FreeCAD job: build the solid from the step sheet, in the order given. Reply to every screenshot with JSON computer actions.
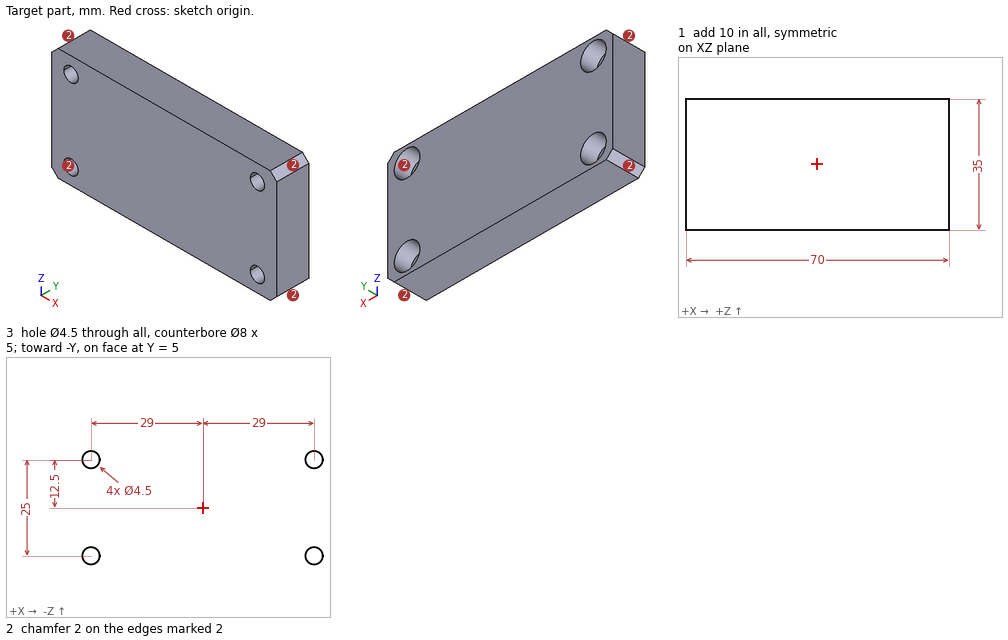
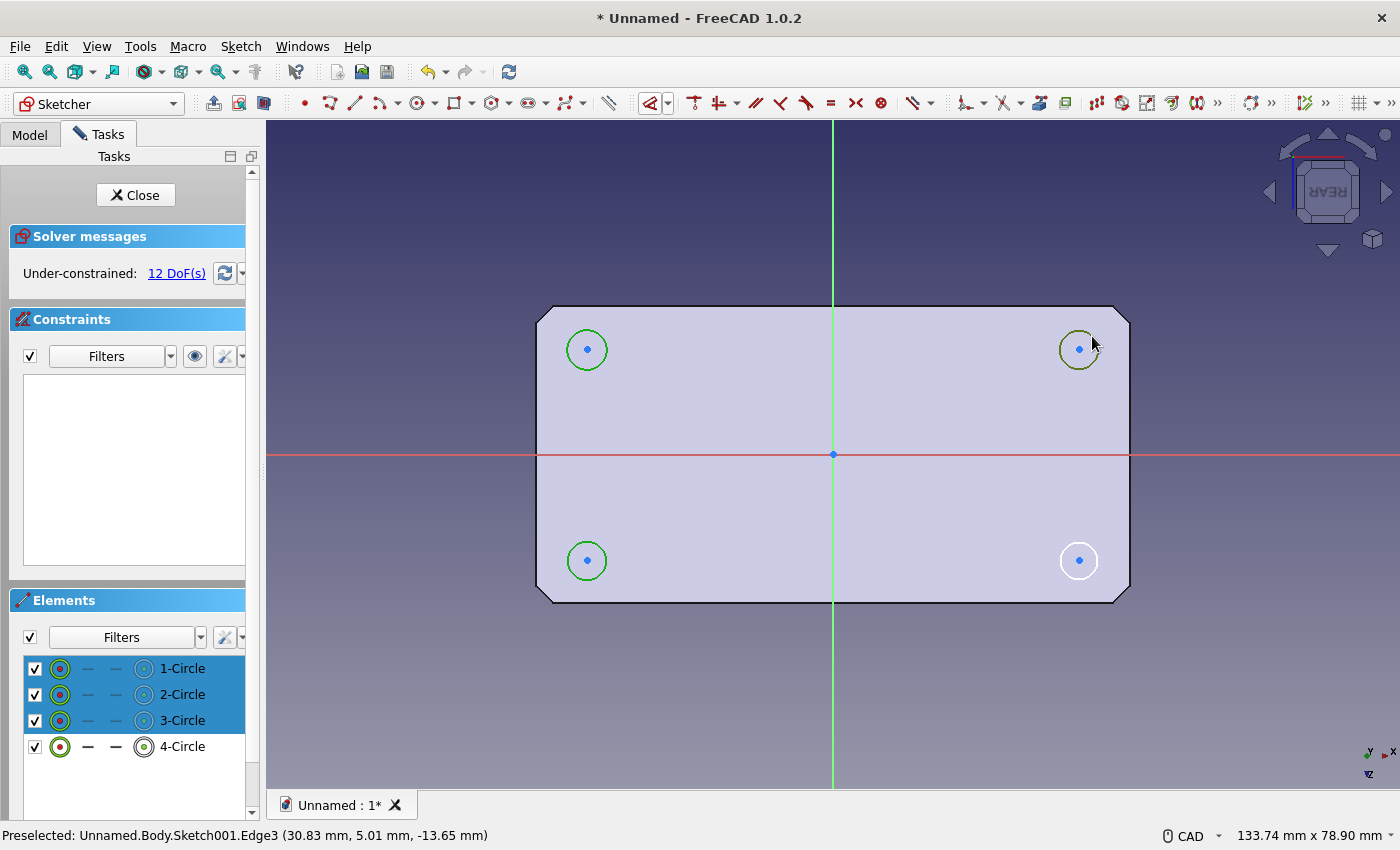
{"action": "left_click", "coordinate": [1092, 548]}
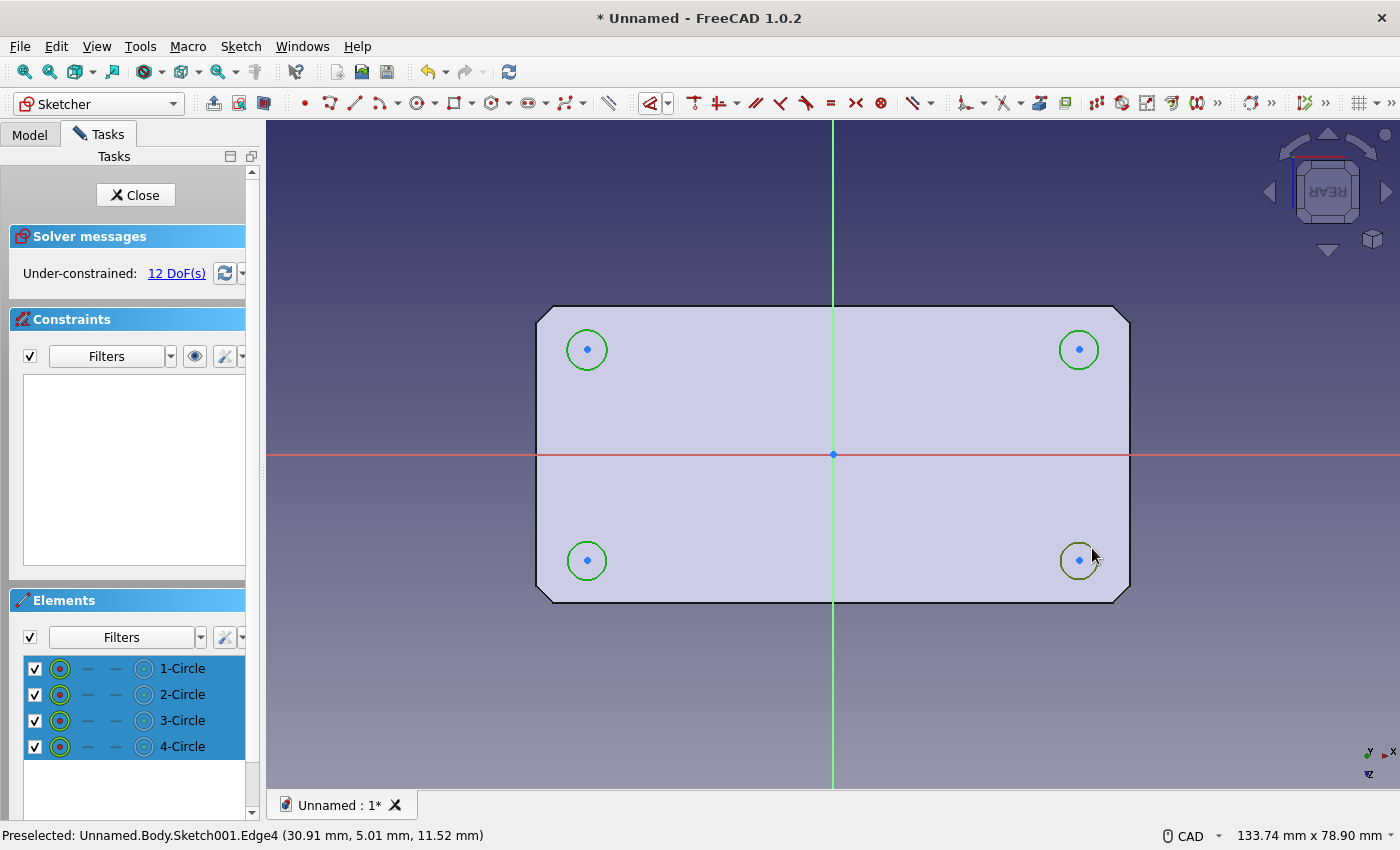
{"action": "left_click", "coordinate": [831, 104]}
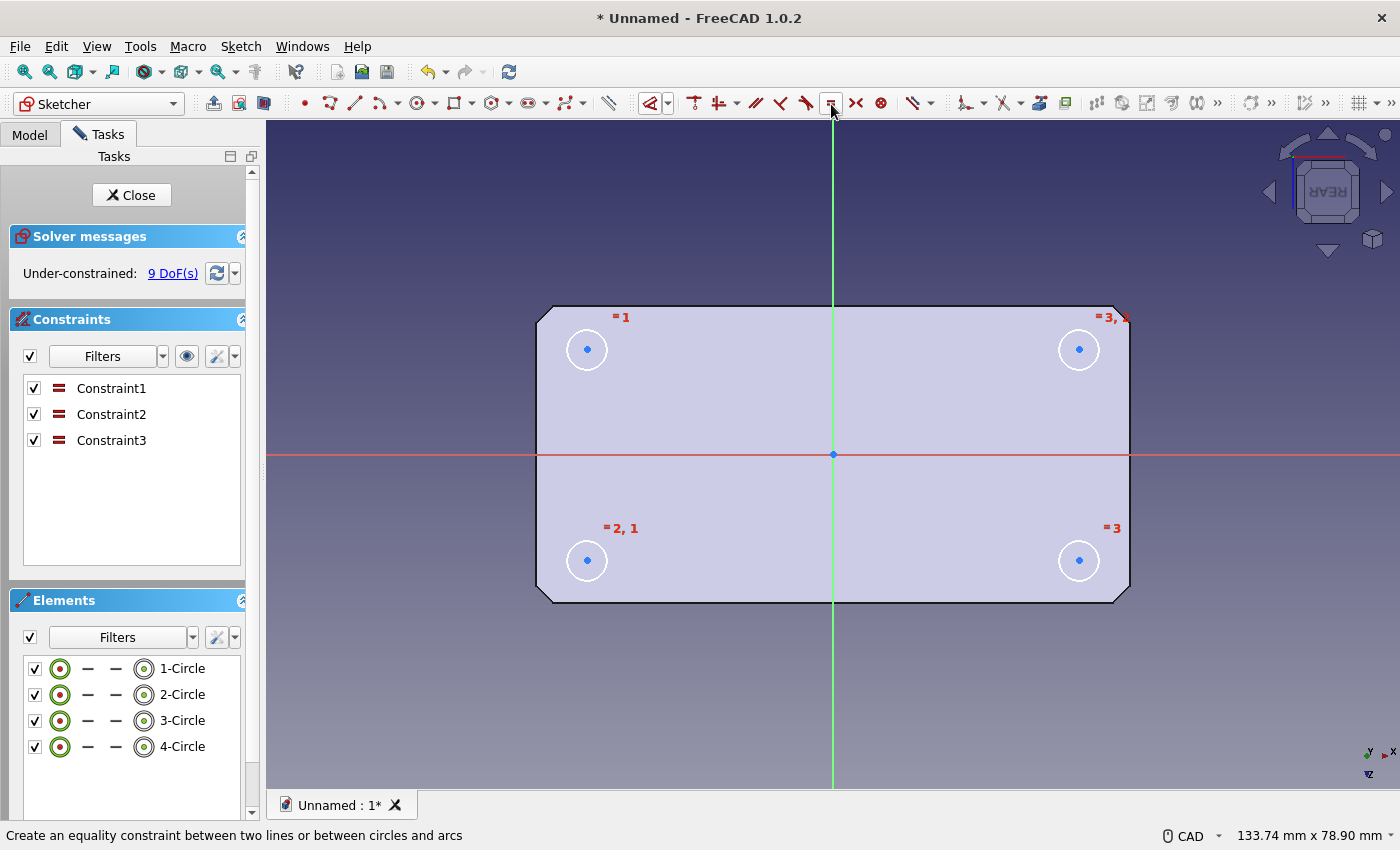
{"action": "left_click", "coordinate": [587, 350]}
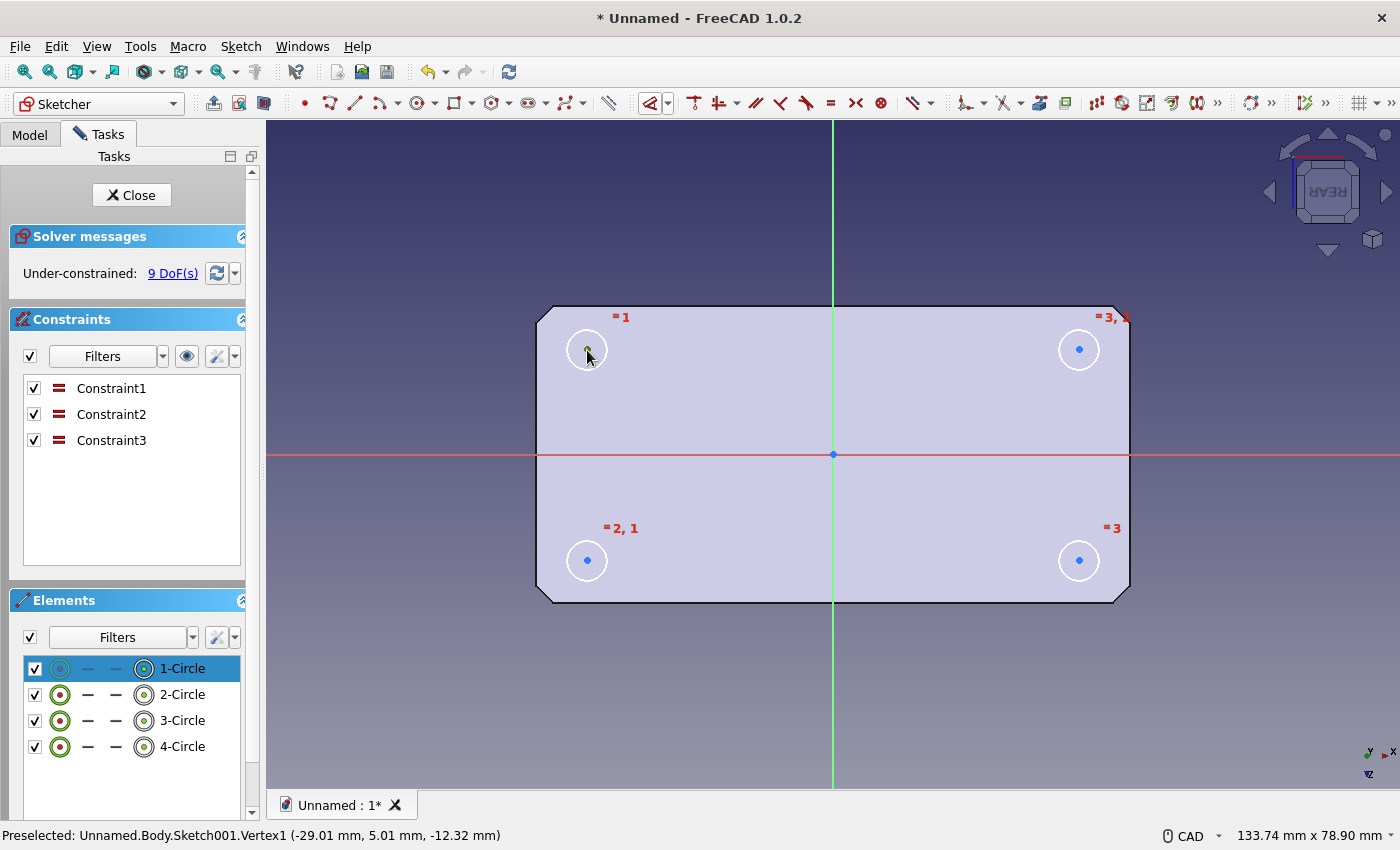
{"action": "left_click", "coordinate": [587, 561]}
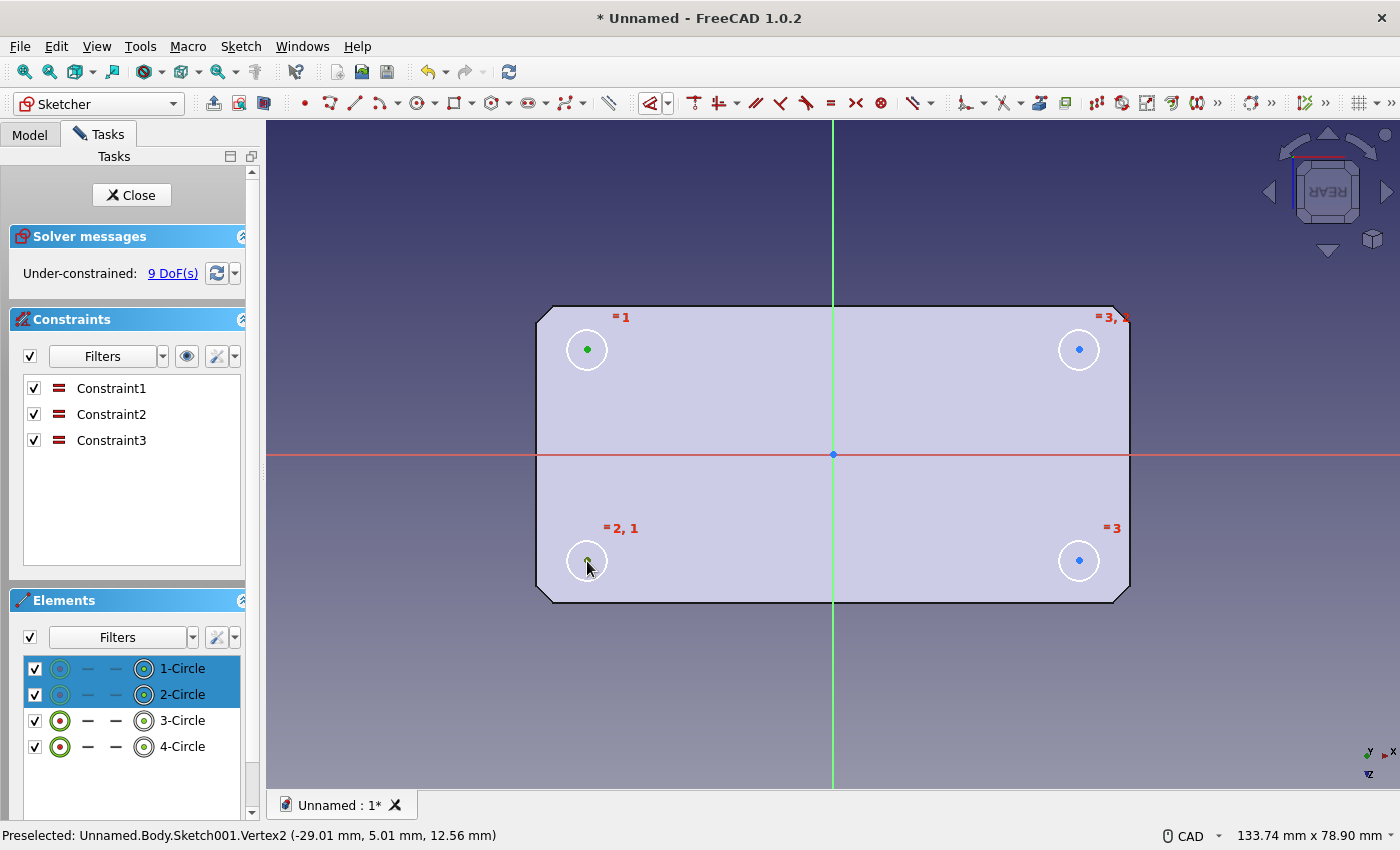
{"action": "left_click", "coordinate": [736, 104]}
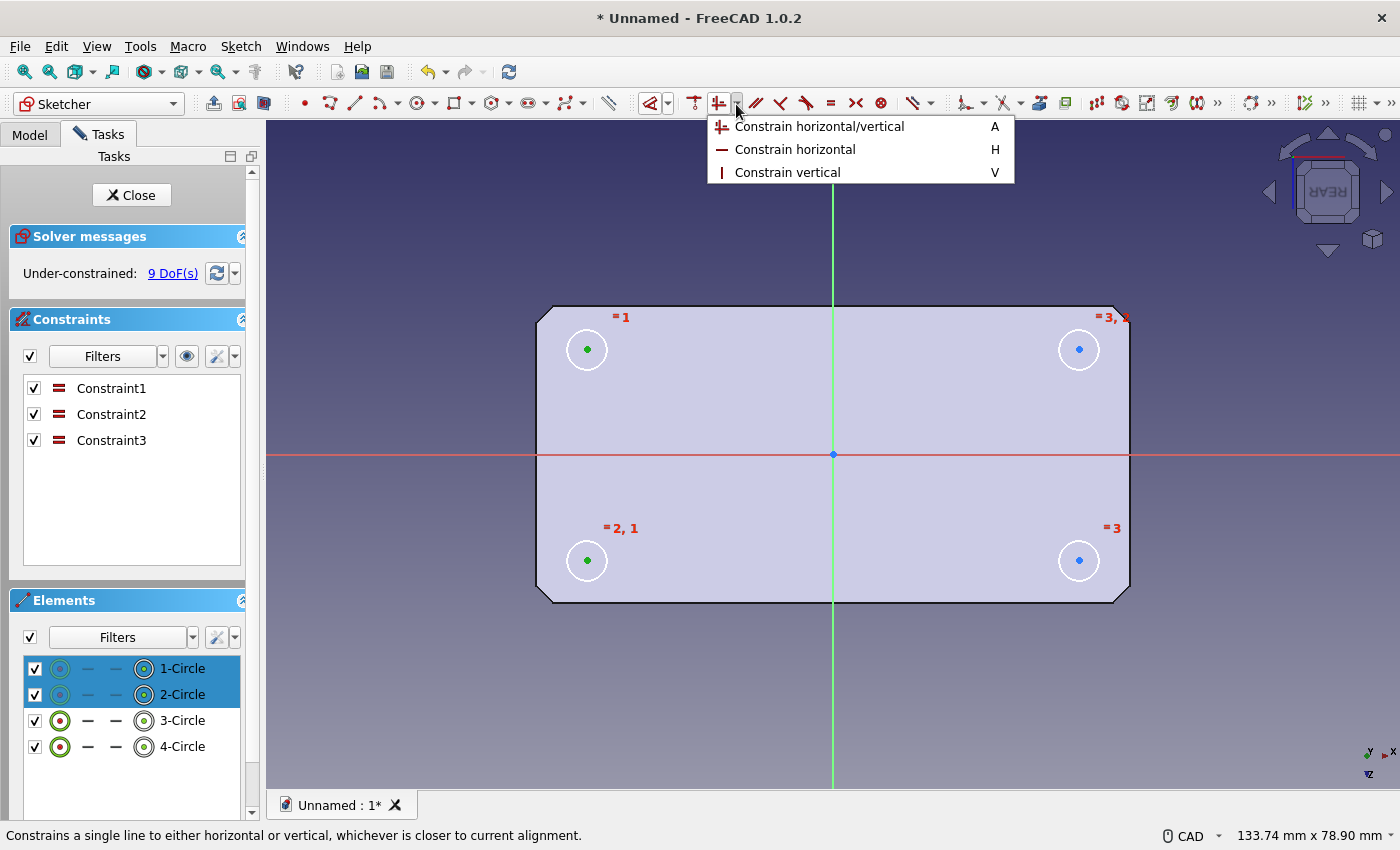
{"action": "left_click", "coordinate": [861, 172]}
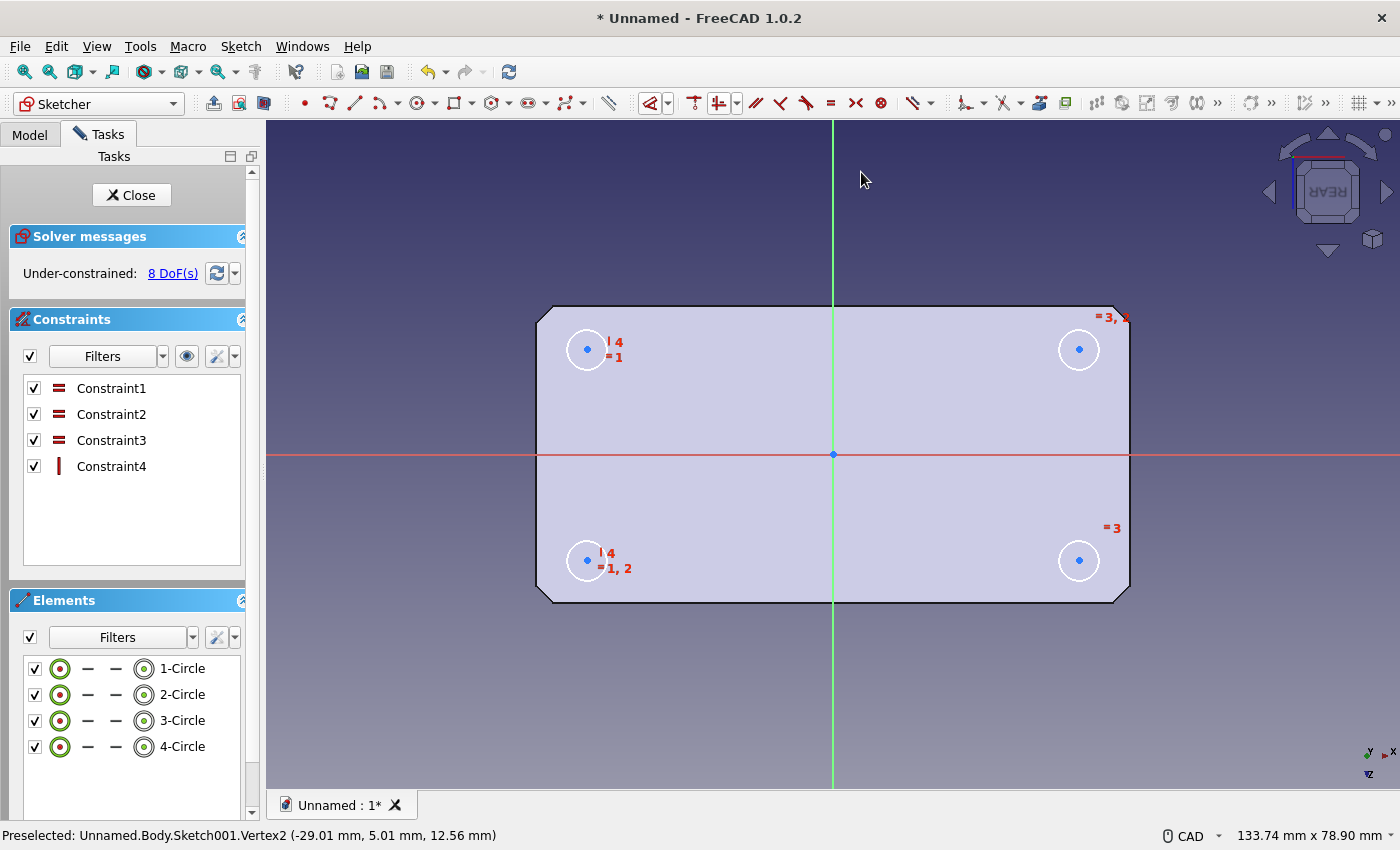
{"action": "left_click", "coordinate": [587, 350]}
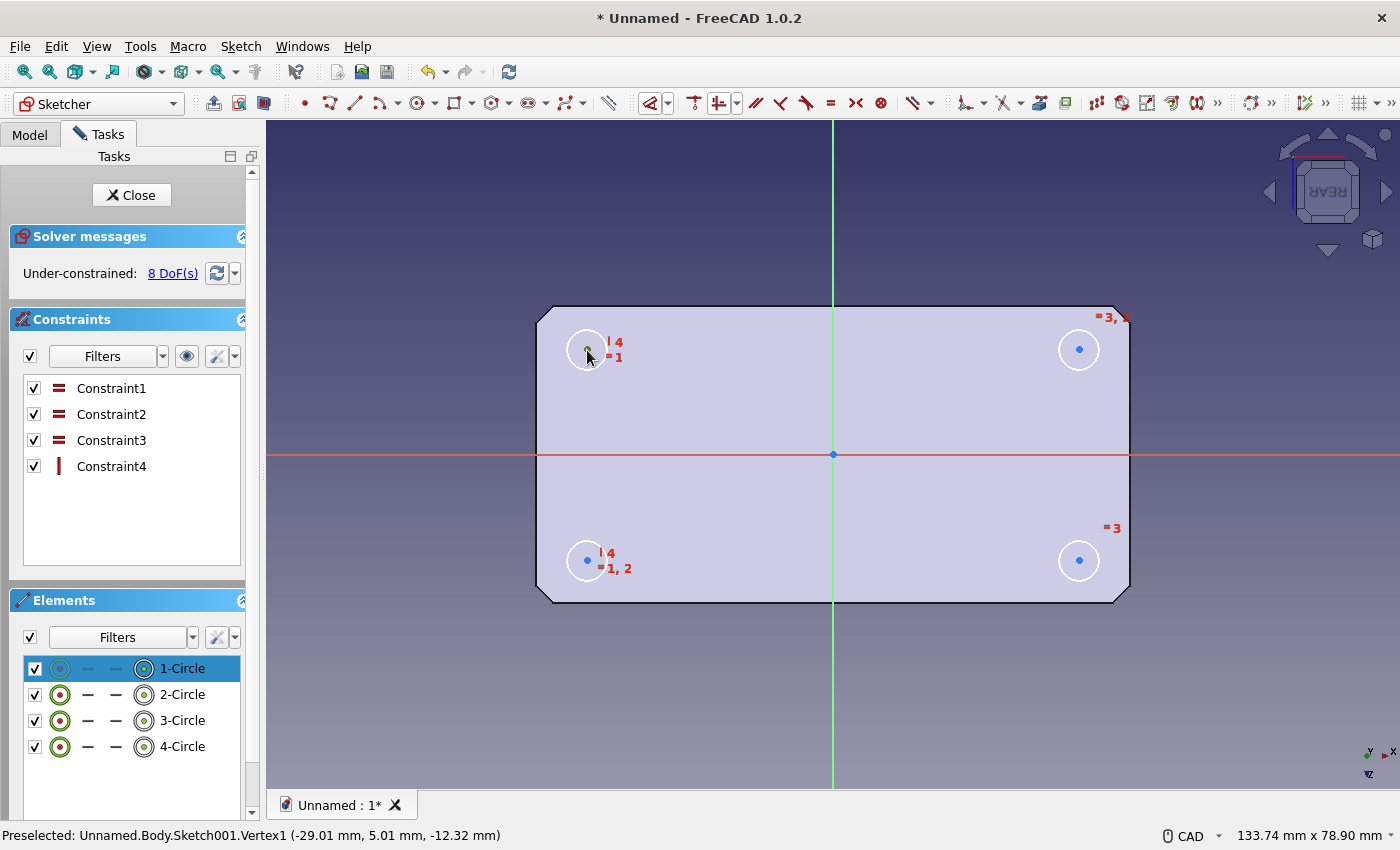
{"action": "left_click", "coordinate": [1079, 350]}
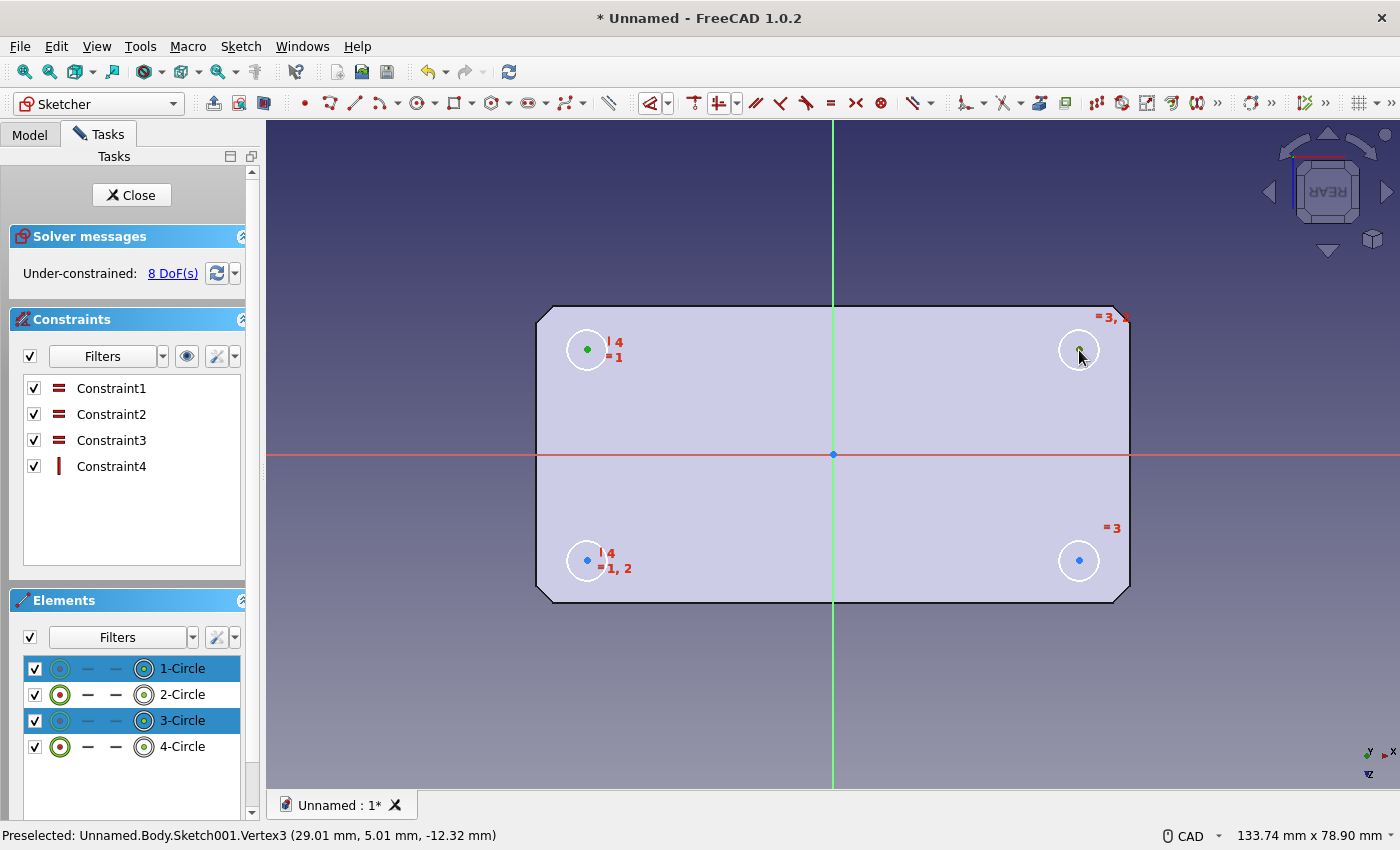
{"action": "left_click", "coordinate": [736, 104]}